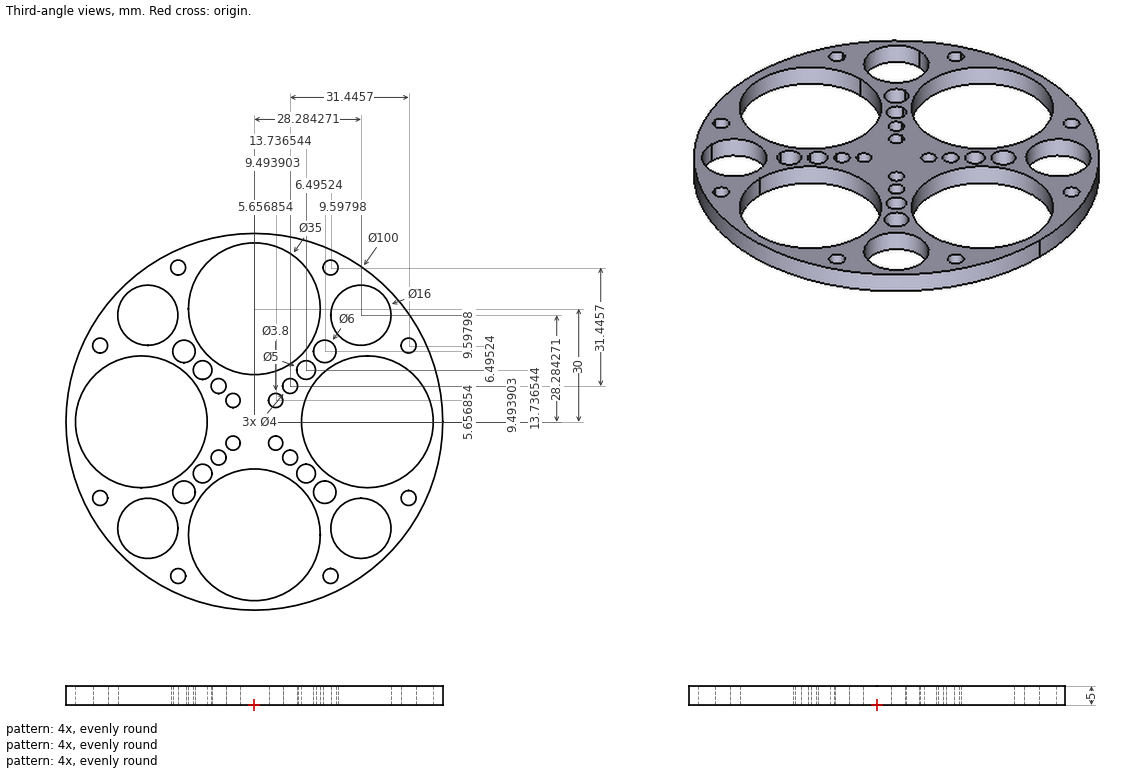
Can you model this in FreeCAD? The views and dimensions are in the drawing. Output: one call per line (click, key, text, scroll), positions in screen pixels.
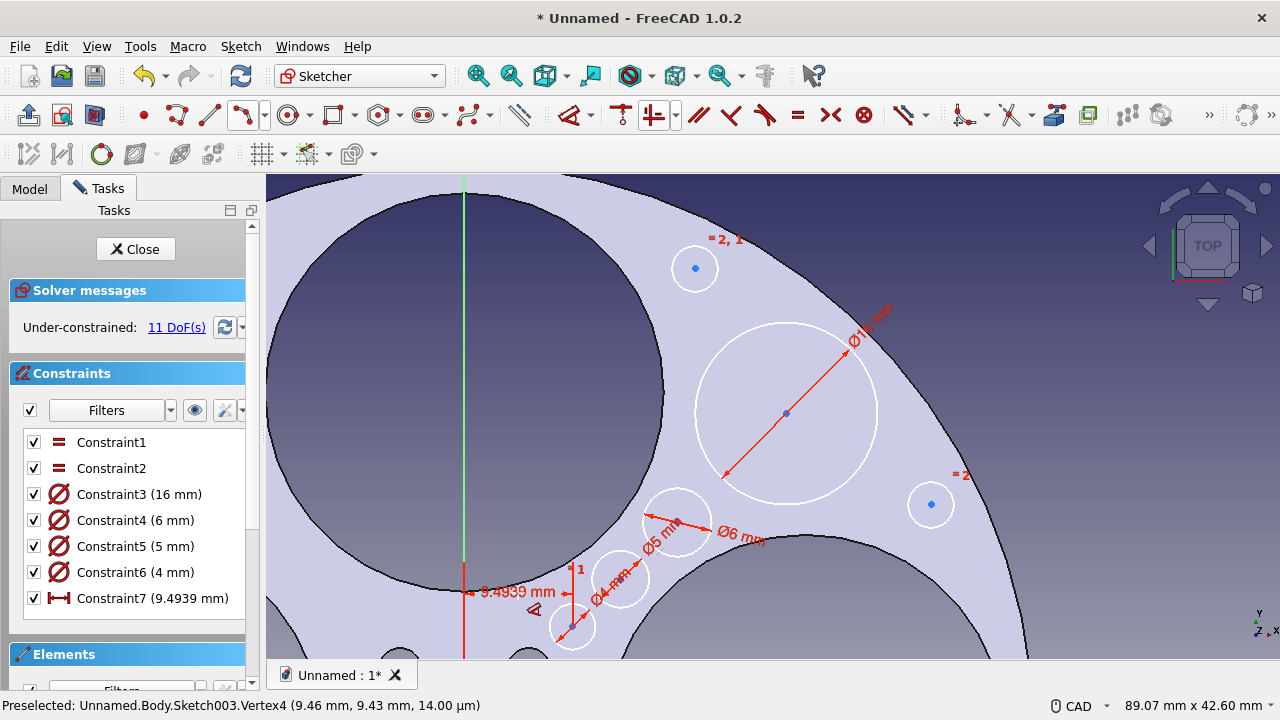
click(573, 627)
click(430, 629)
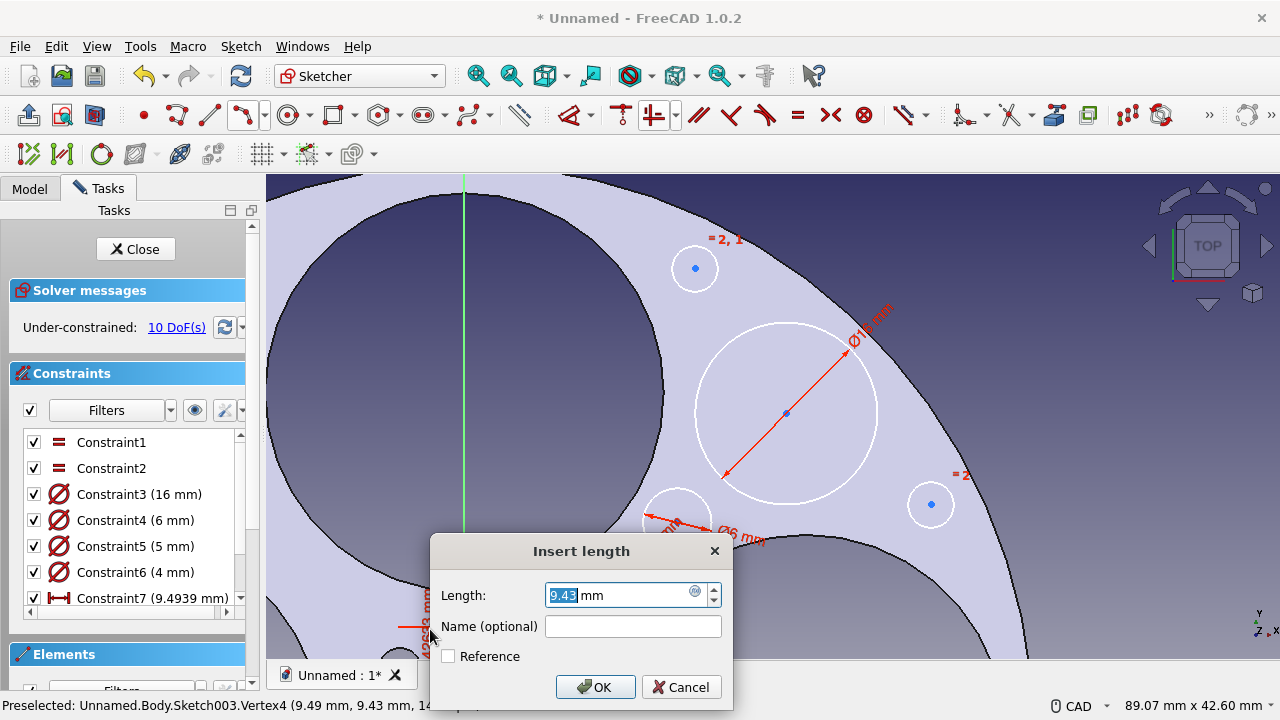
text(9.493903)
key(Return)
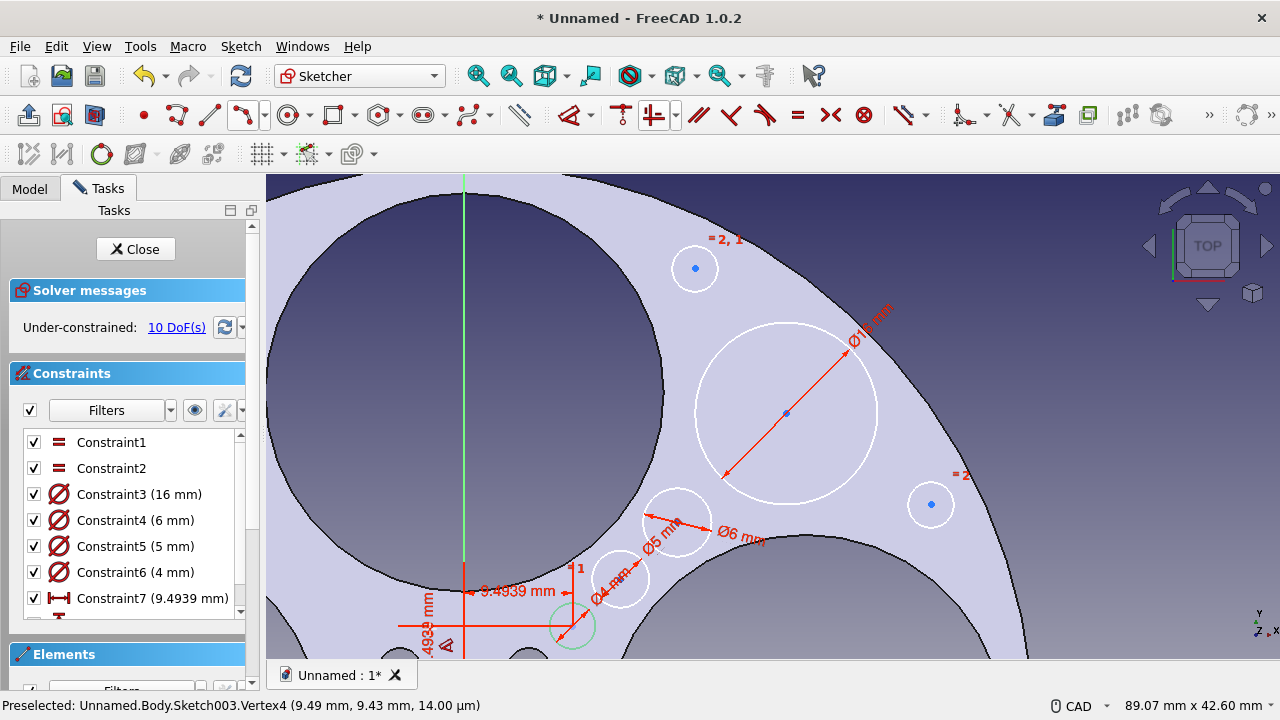
click(786, 414)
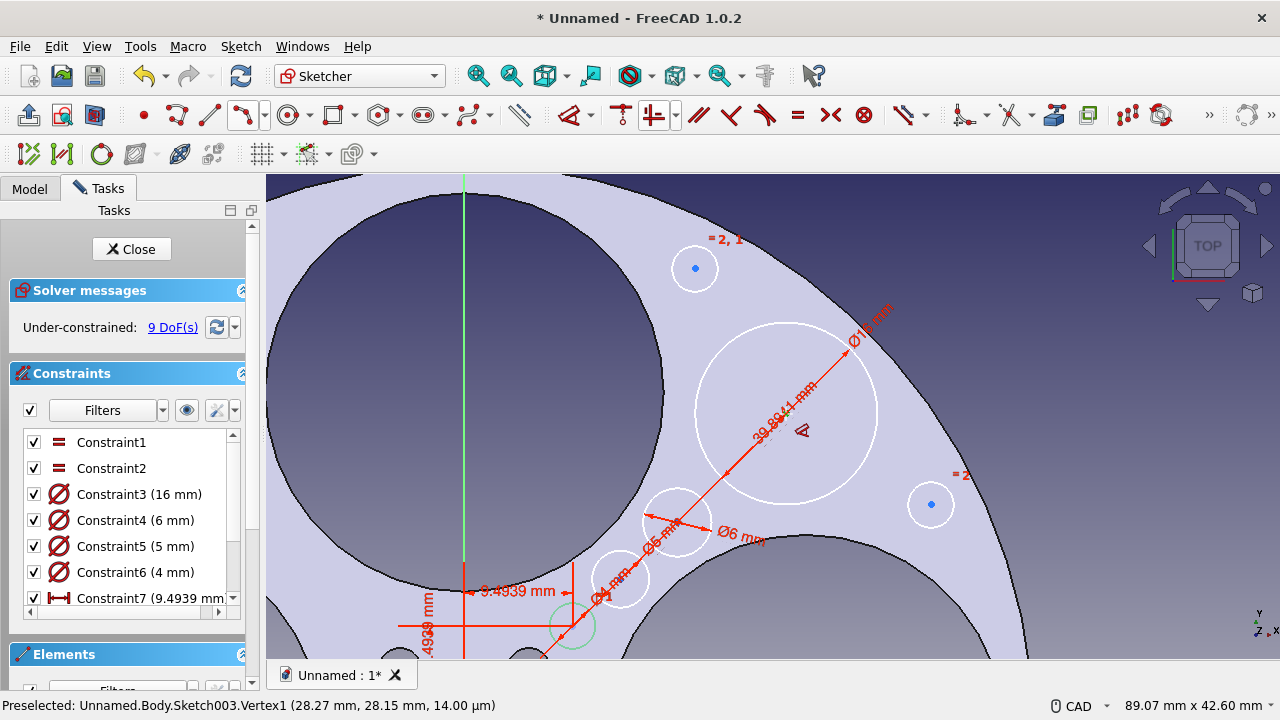
click(677, 523)
click(732, 380)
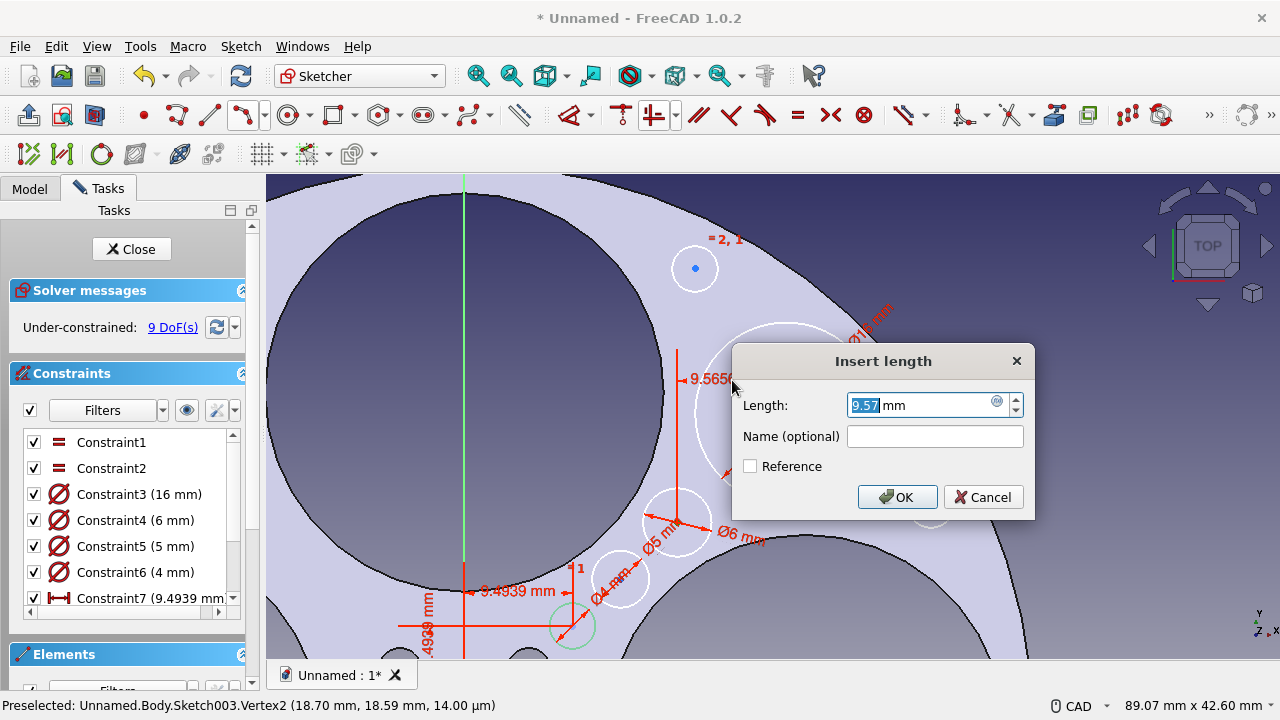
text(9.59798)
key(Return)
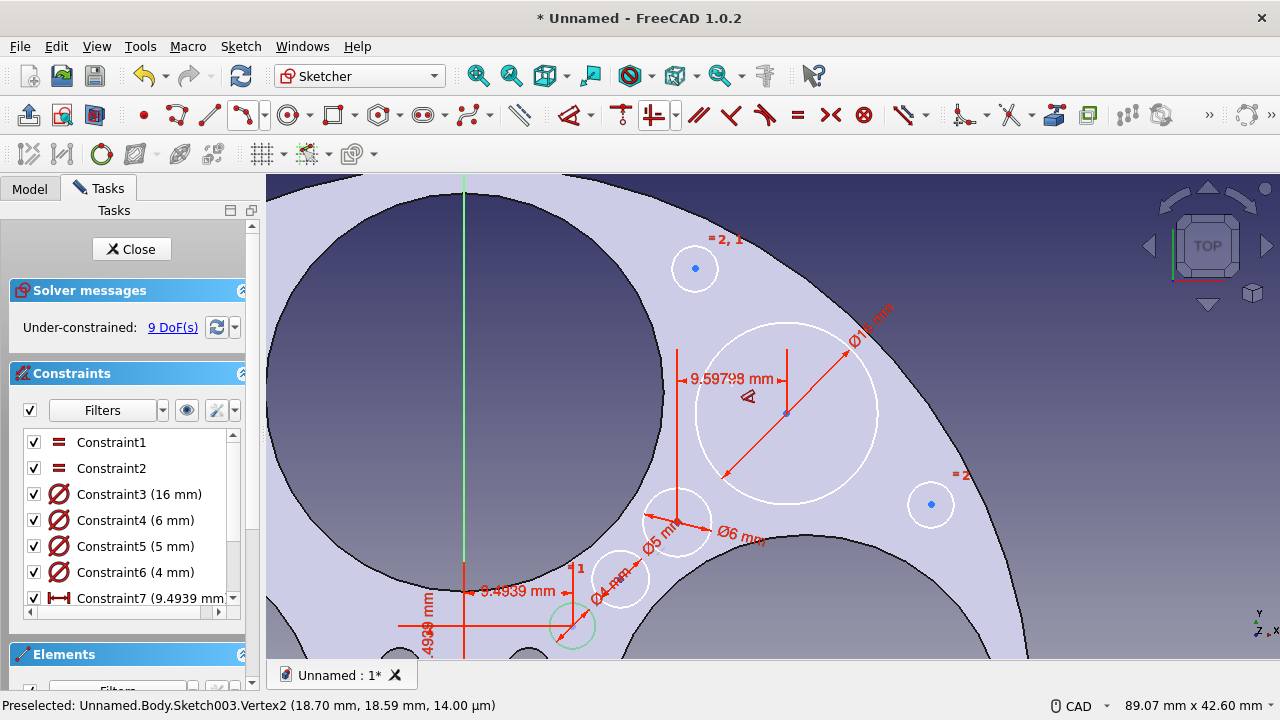
click(787, 414)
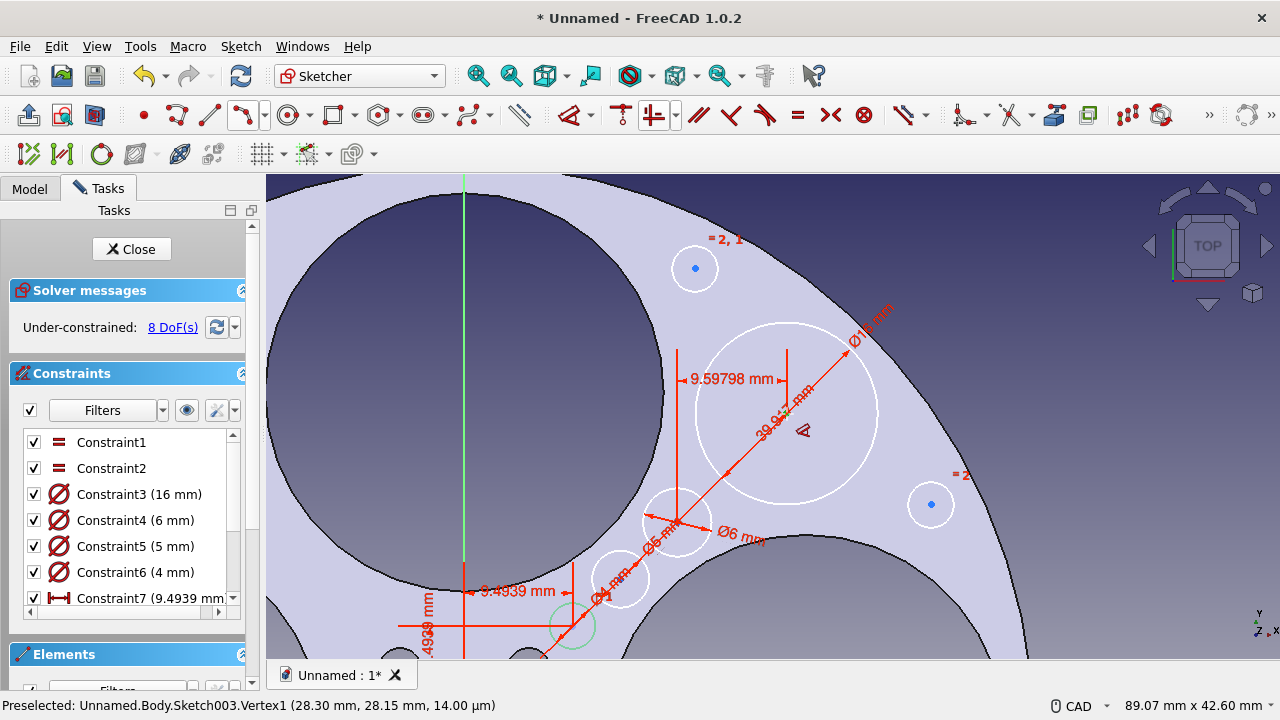
click(677, 523)
click(821, 468)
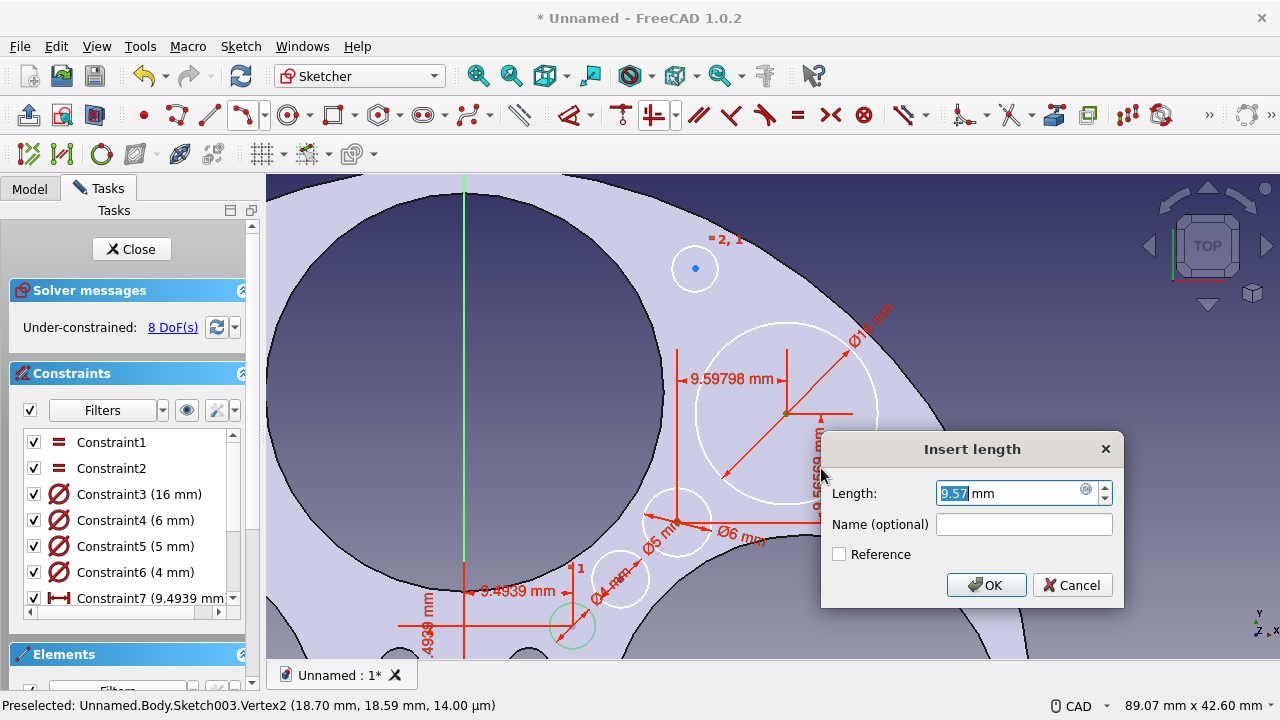
text(9.59798)
key(Return)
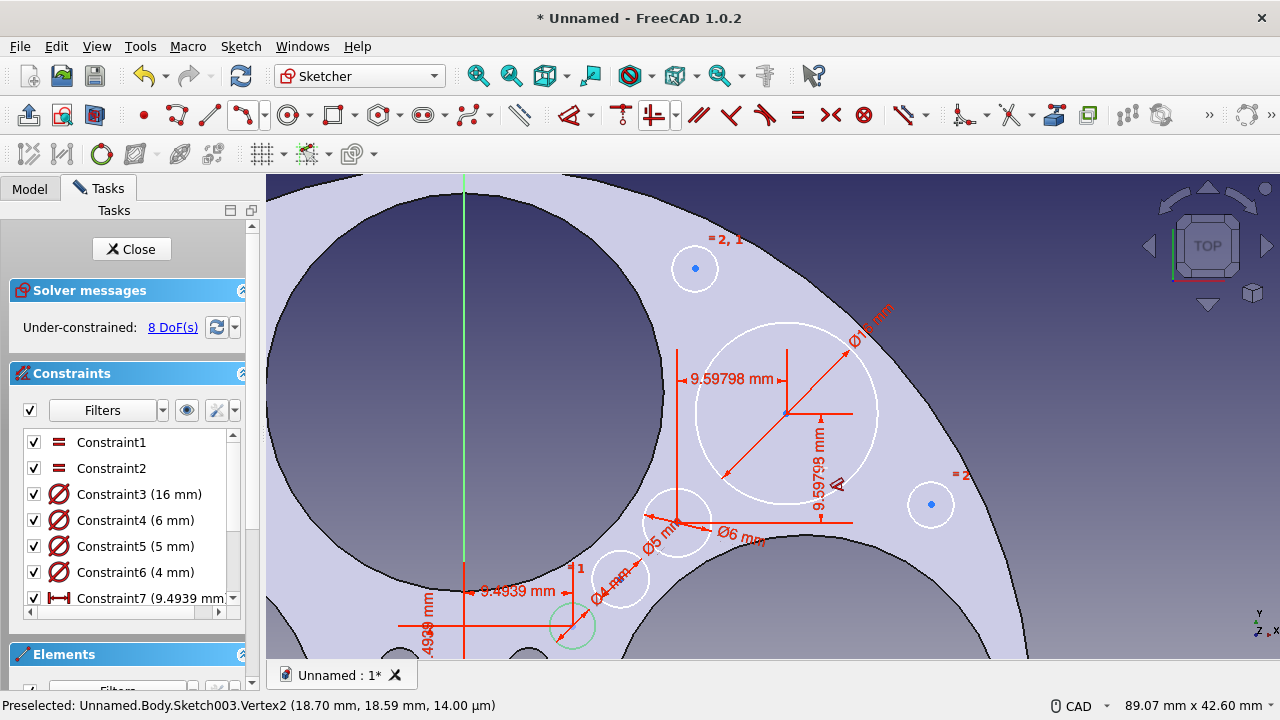
click(621, 579)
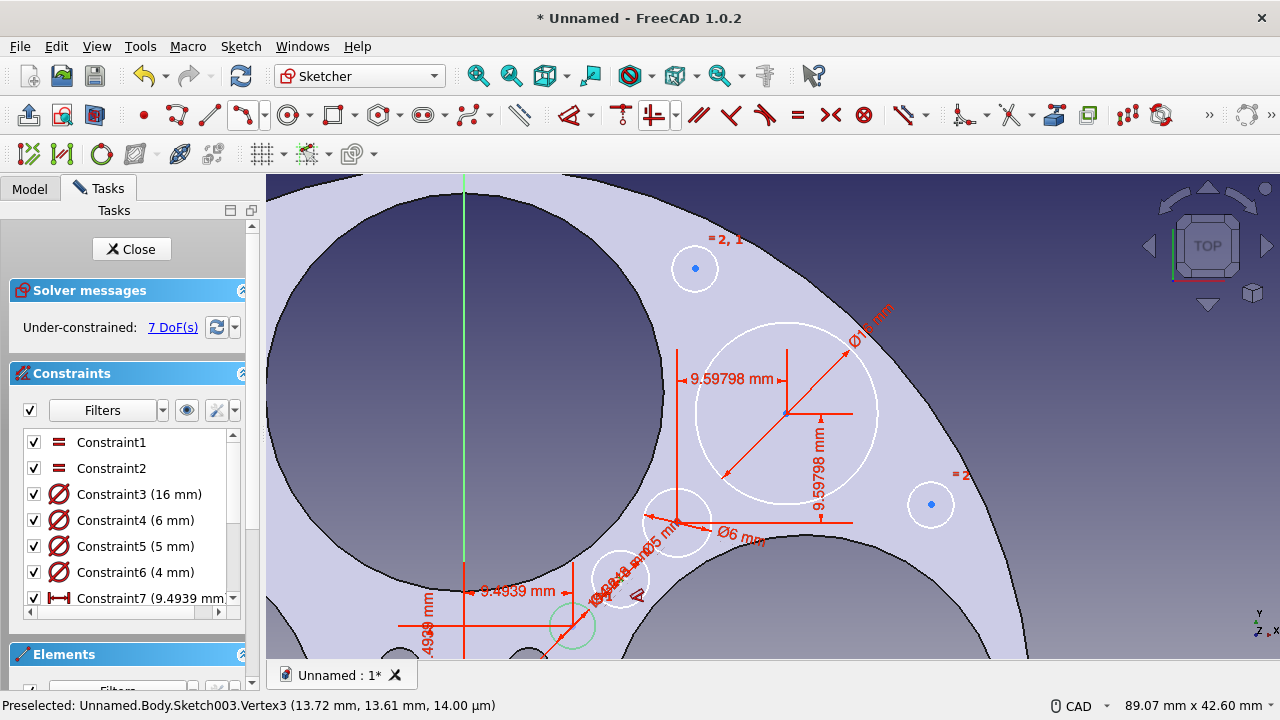
click(695, 269)
click(658, 235)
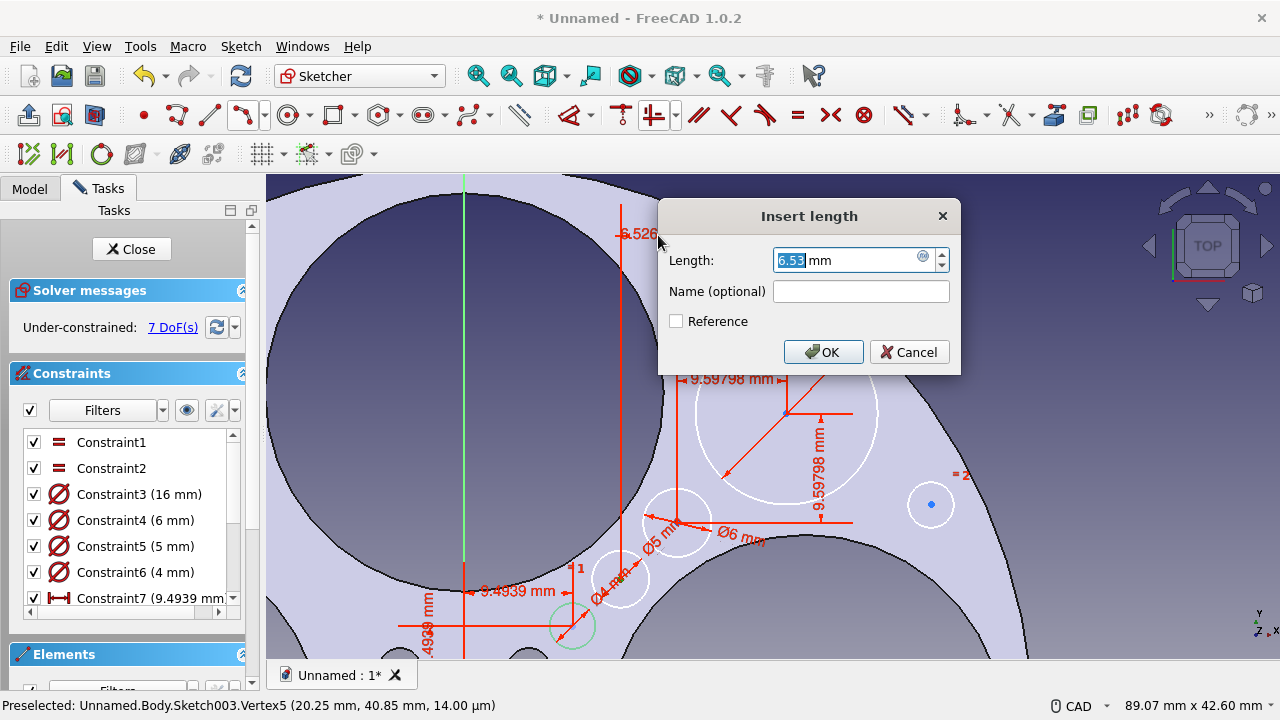
text(6.49524)
key(Return)